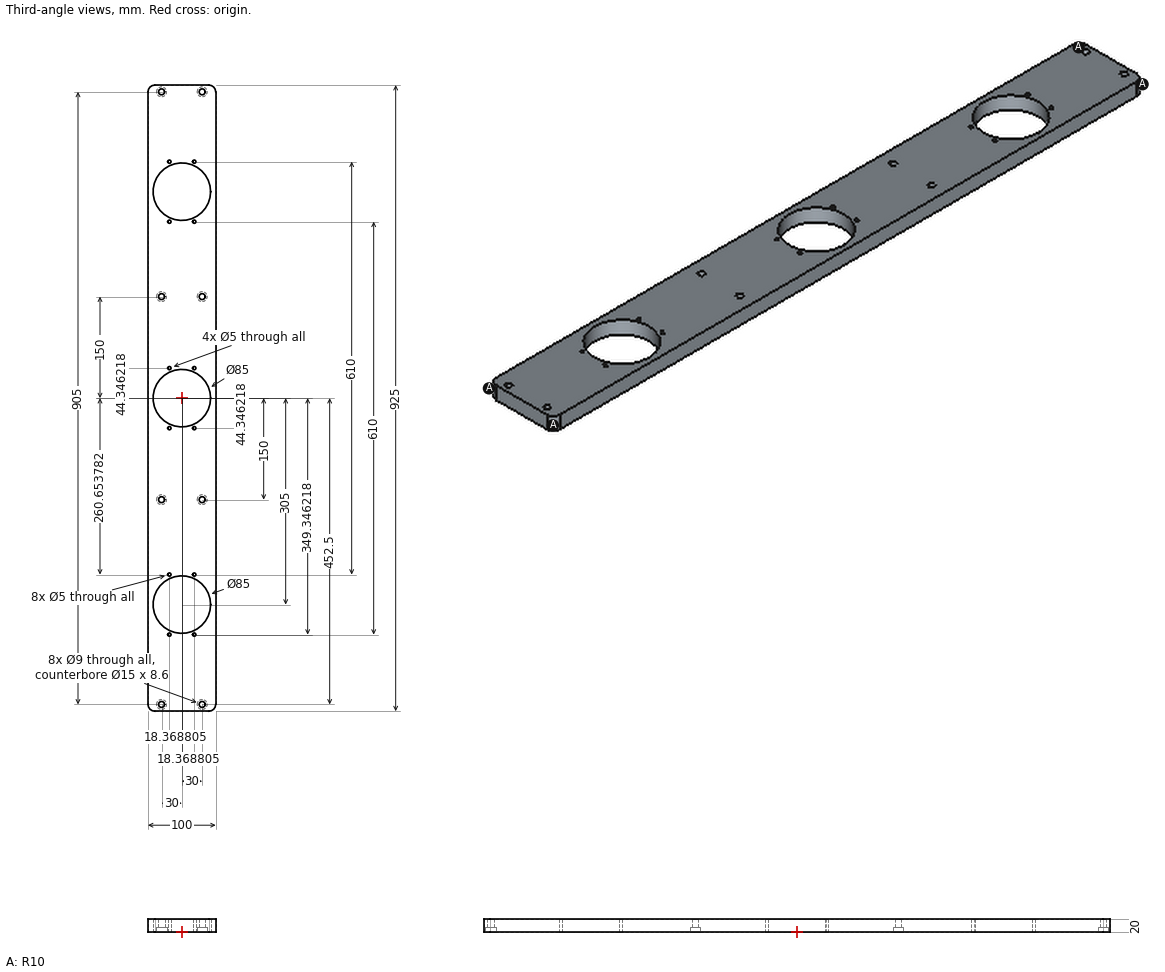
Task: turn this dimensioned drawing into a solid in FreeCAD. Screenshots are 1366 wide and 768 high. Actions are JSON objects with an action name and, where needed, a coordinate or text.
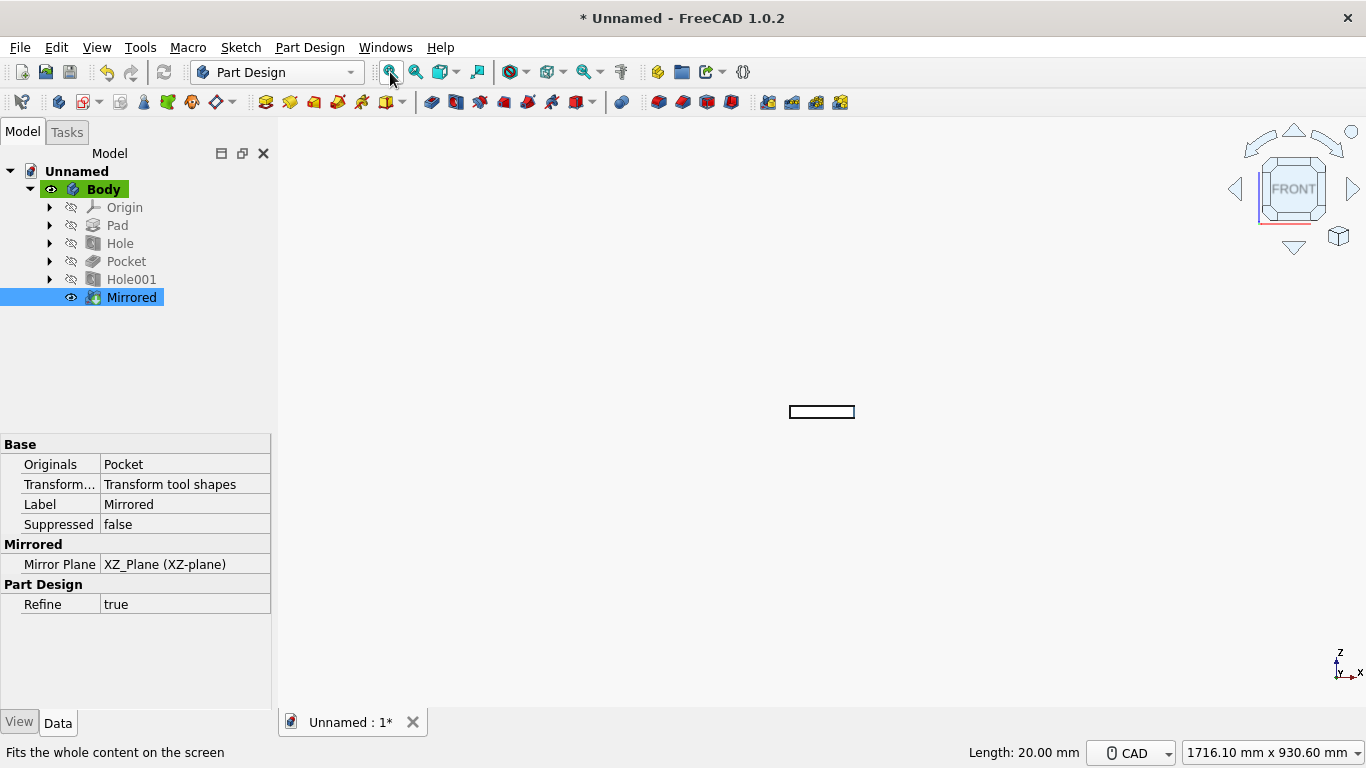
{"action": "left_click", "coordinate": [790, 411], "text": "ctrl"}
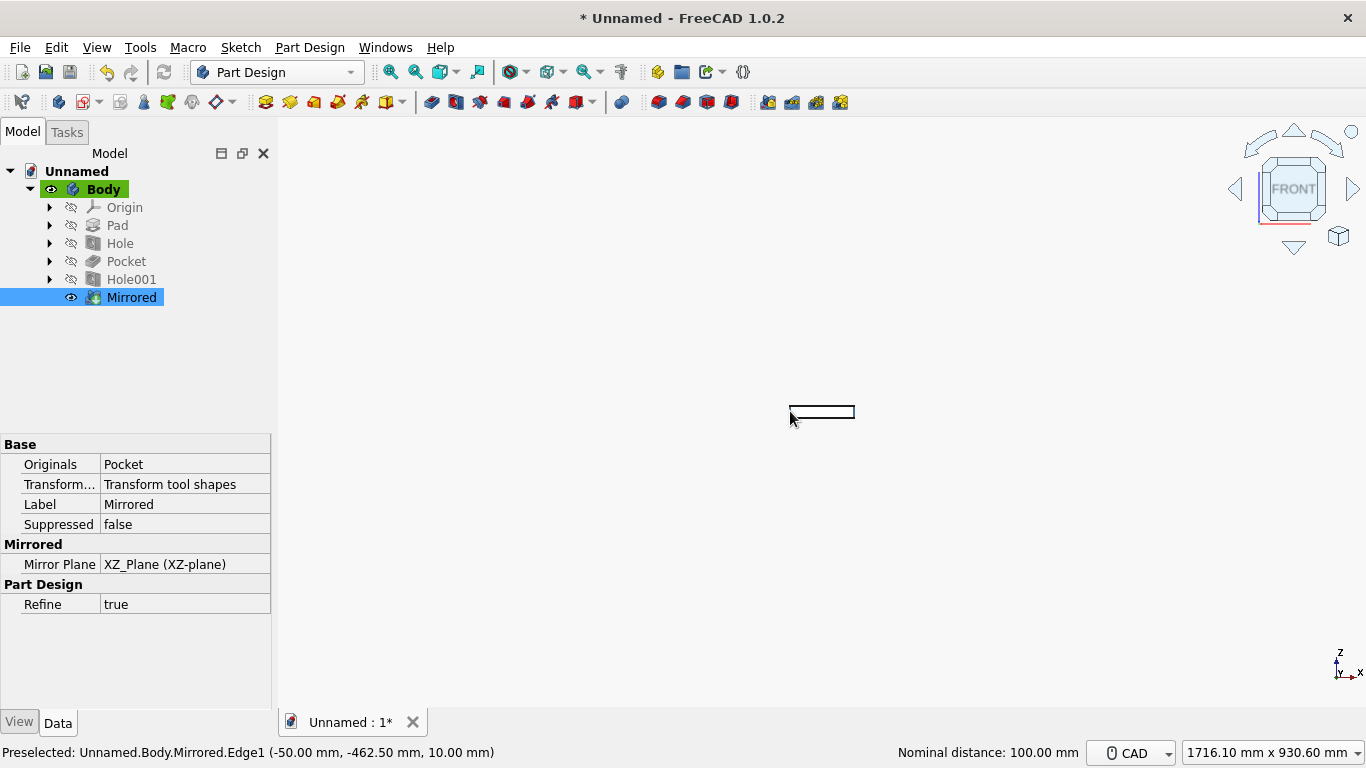
{"action": "scroll", "coordinate": [790, 411], "scroll_direction": "up", "scroll_amount": 6}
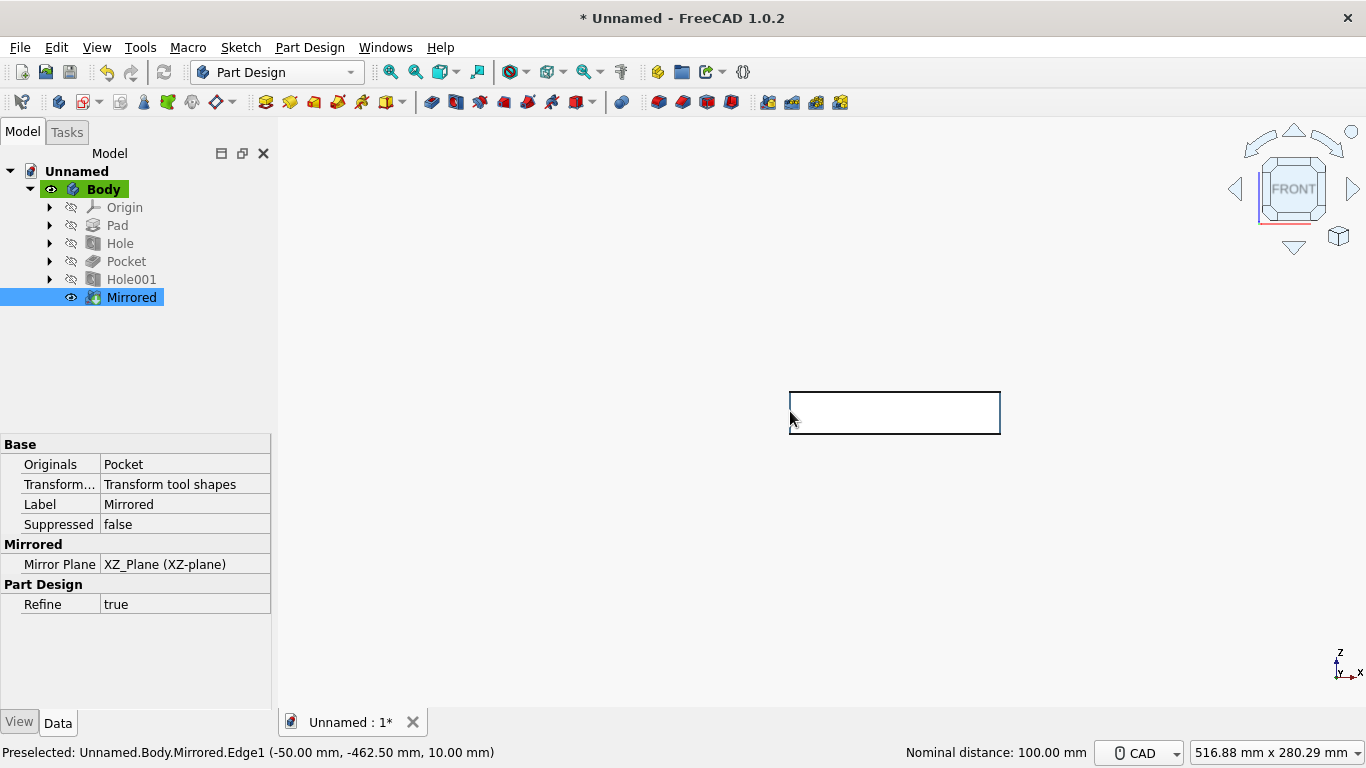
{"action": "key", "text": "v f"}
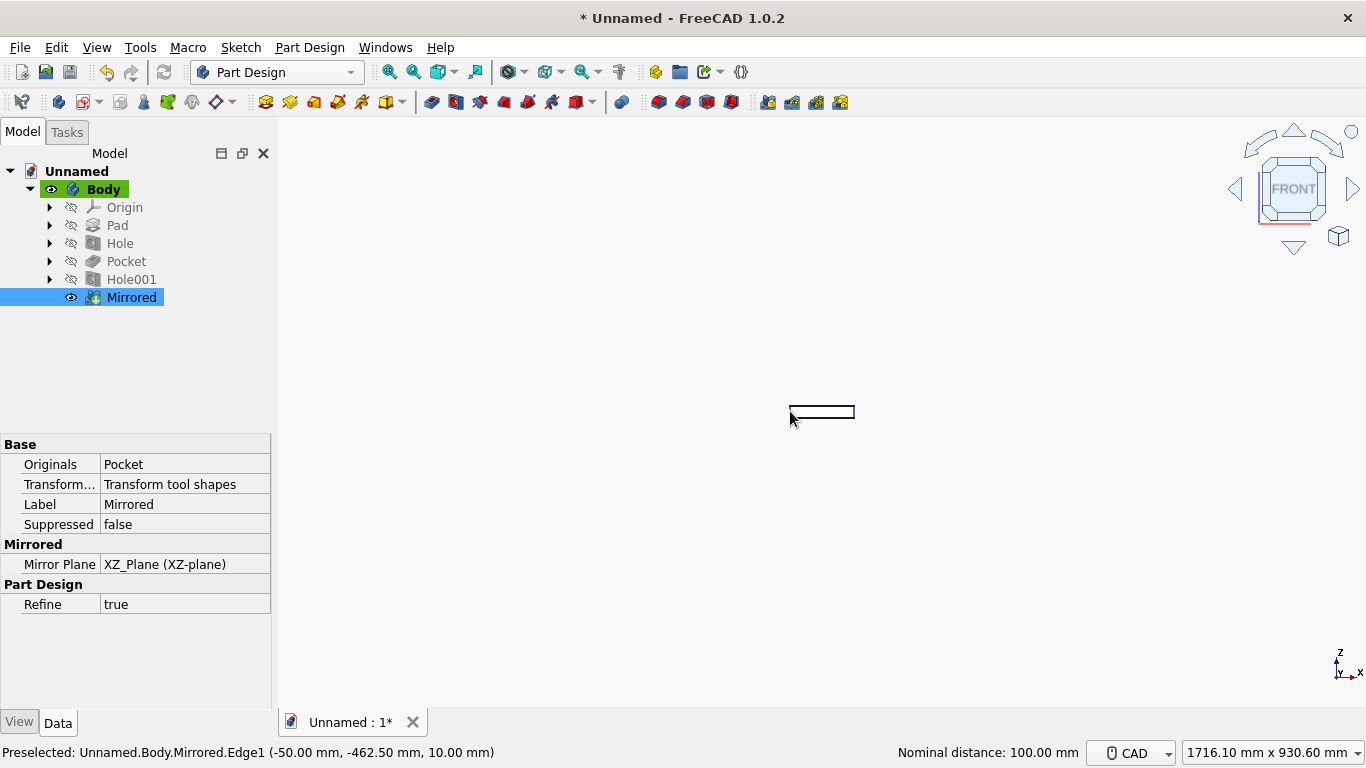
{"action": "key", "text": "3"}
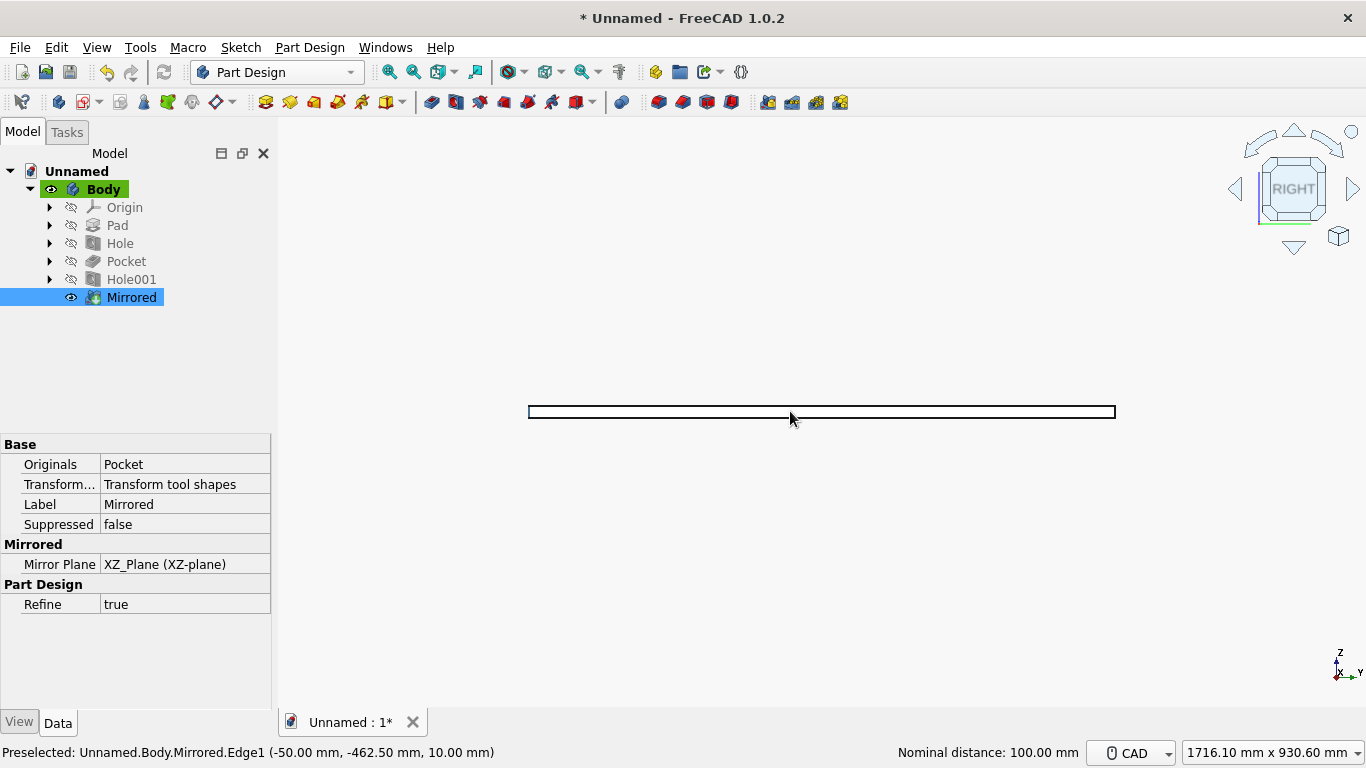
{"action": "left_click", "coordinate": [1115, 411], "text": "ctrl"}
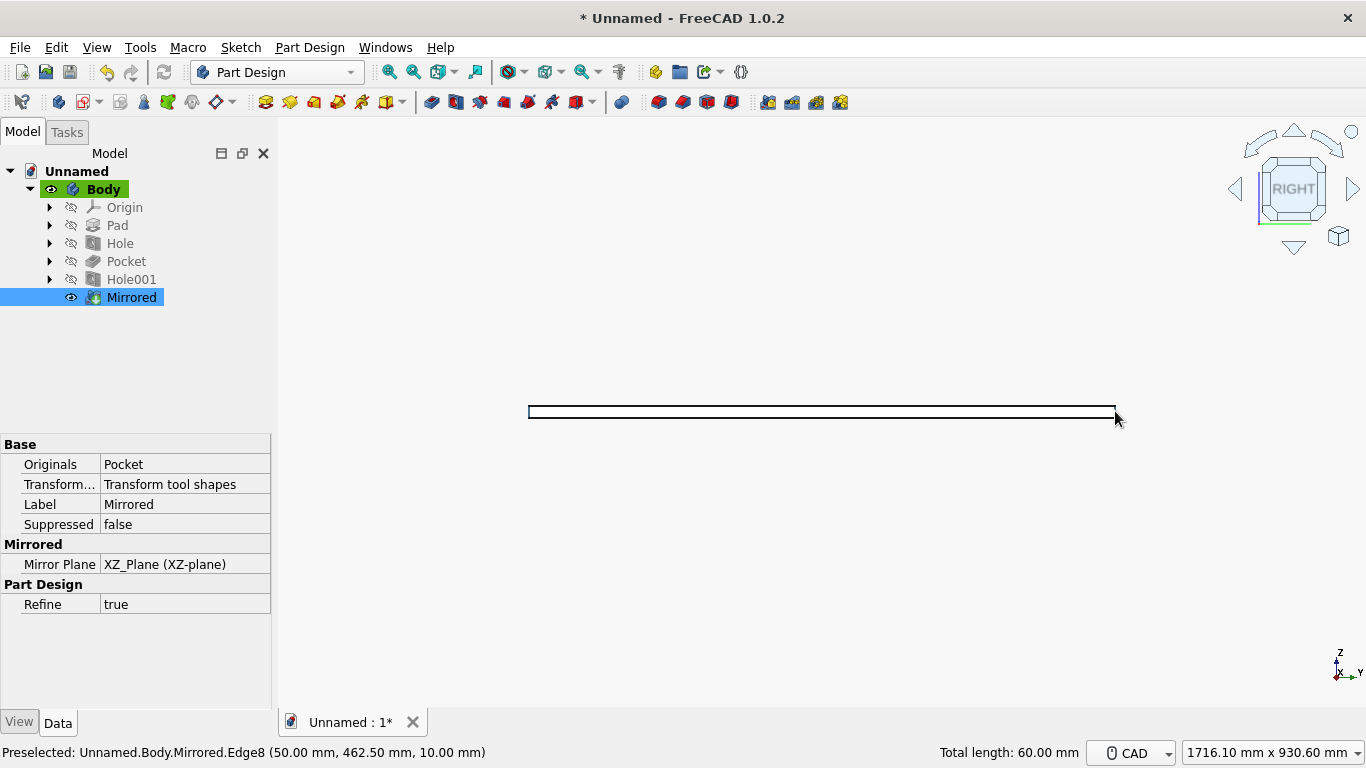
{"action": "scroll", "coordinate": [1115, 411], "scroll_direction": "up", "scroll_amount": 6}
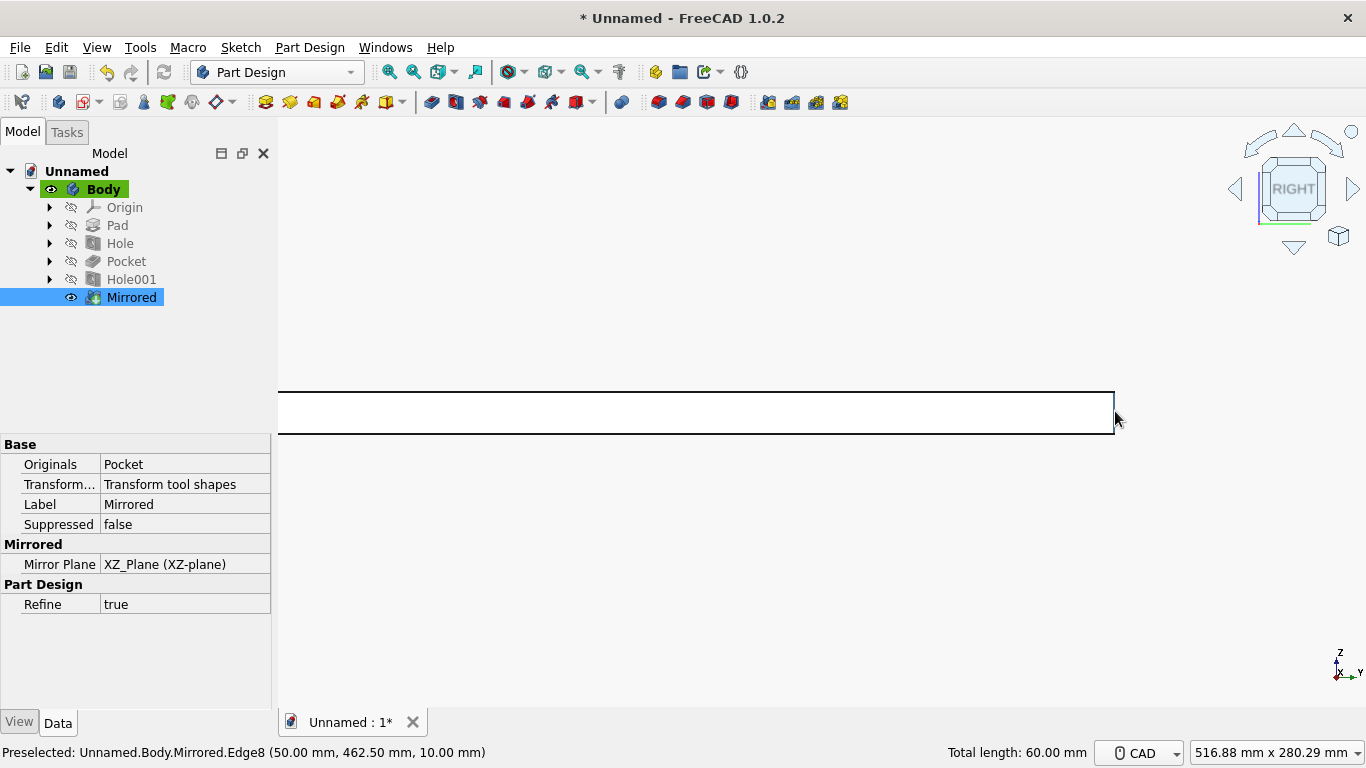
{"action": "key", "text": "v f"}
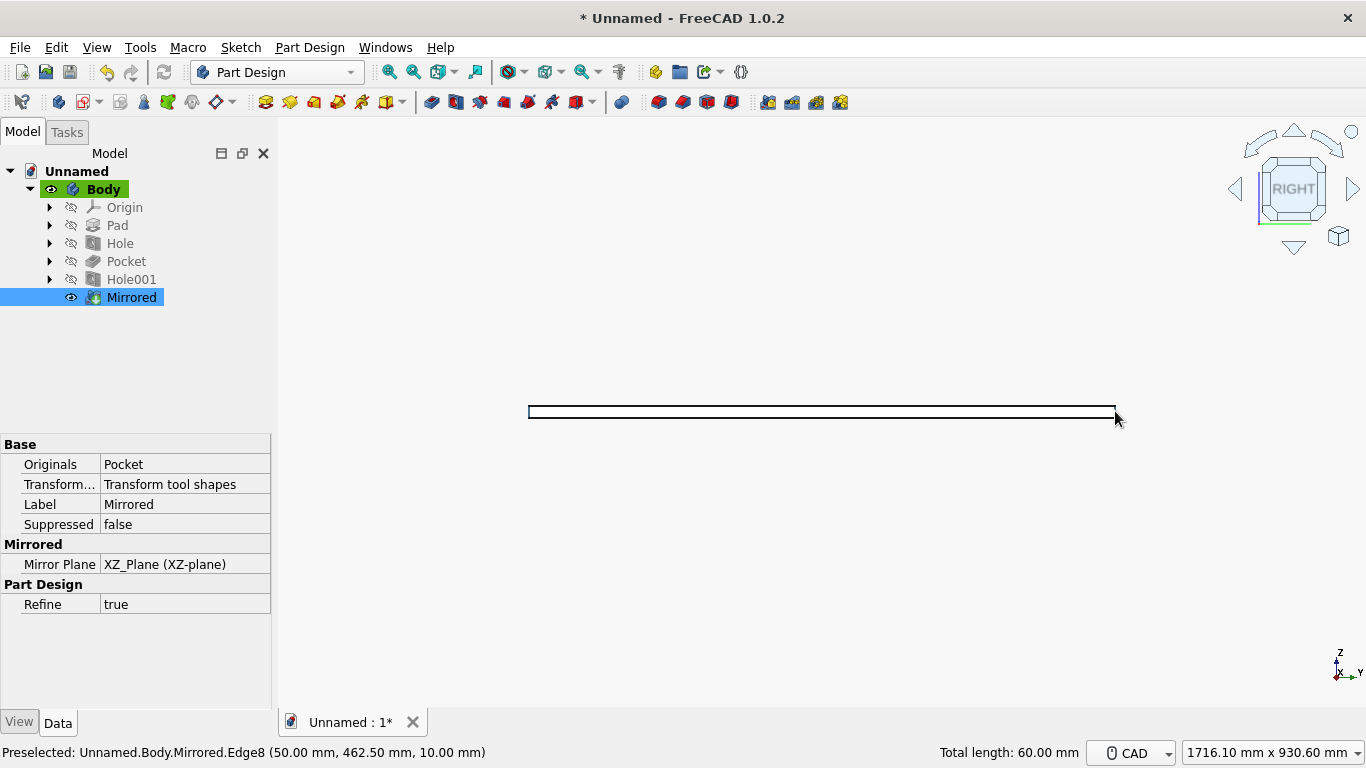
{"action": "key", "text": "5"}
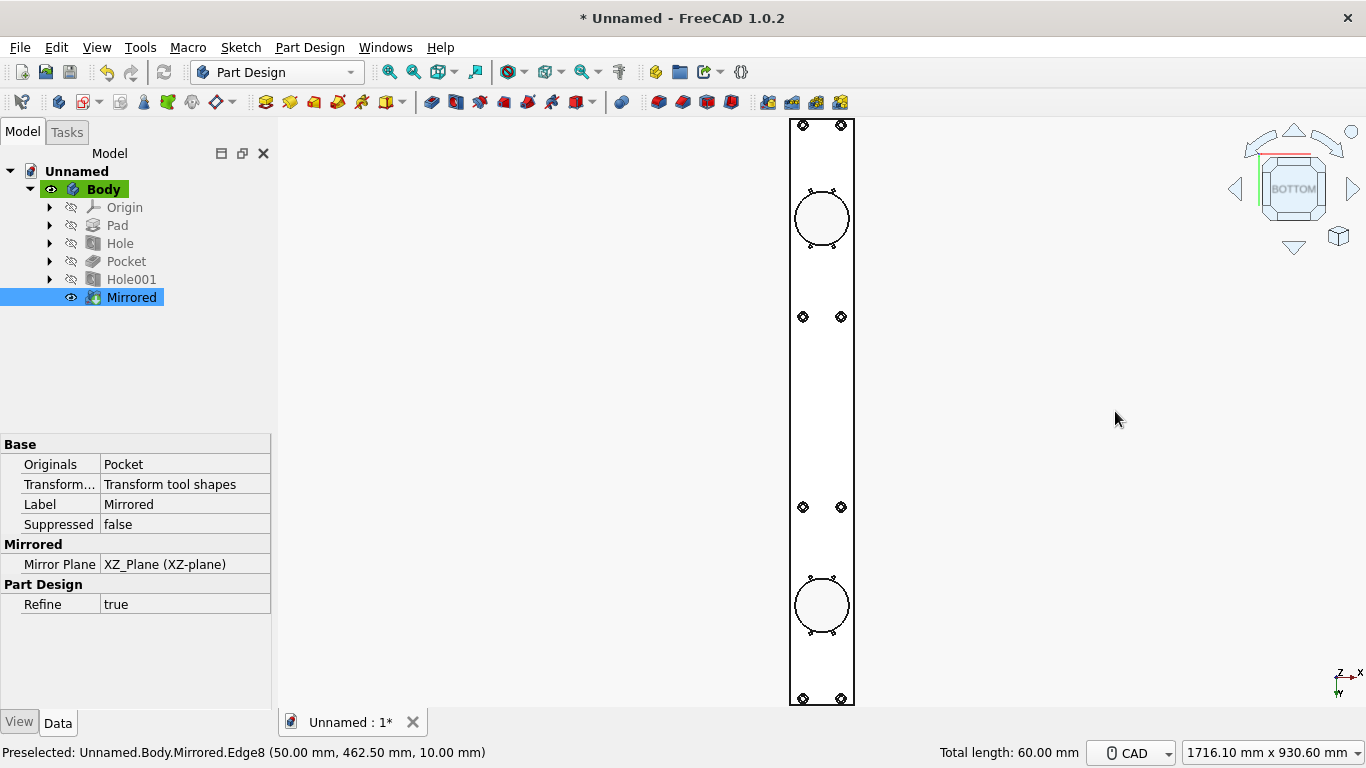
{"action": "key", "text": "4"}